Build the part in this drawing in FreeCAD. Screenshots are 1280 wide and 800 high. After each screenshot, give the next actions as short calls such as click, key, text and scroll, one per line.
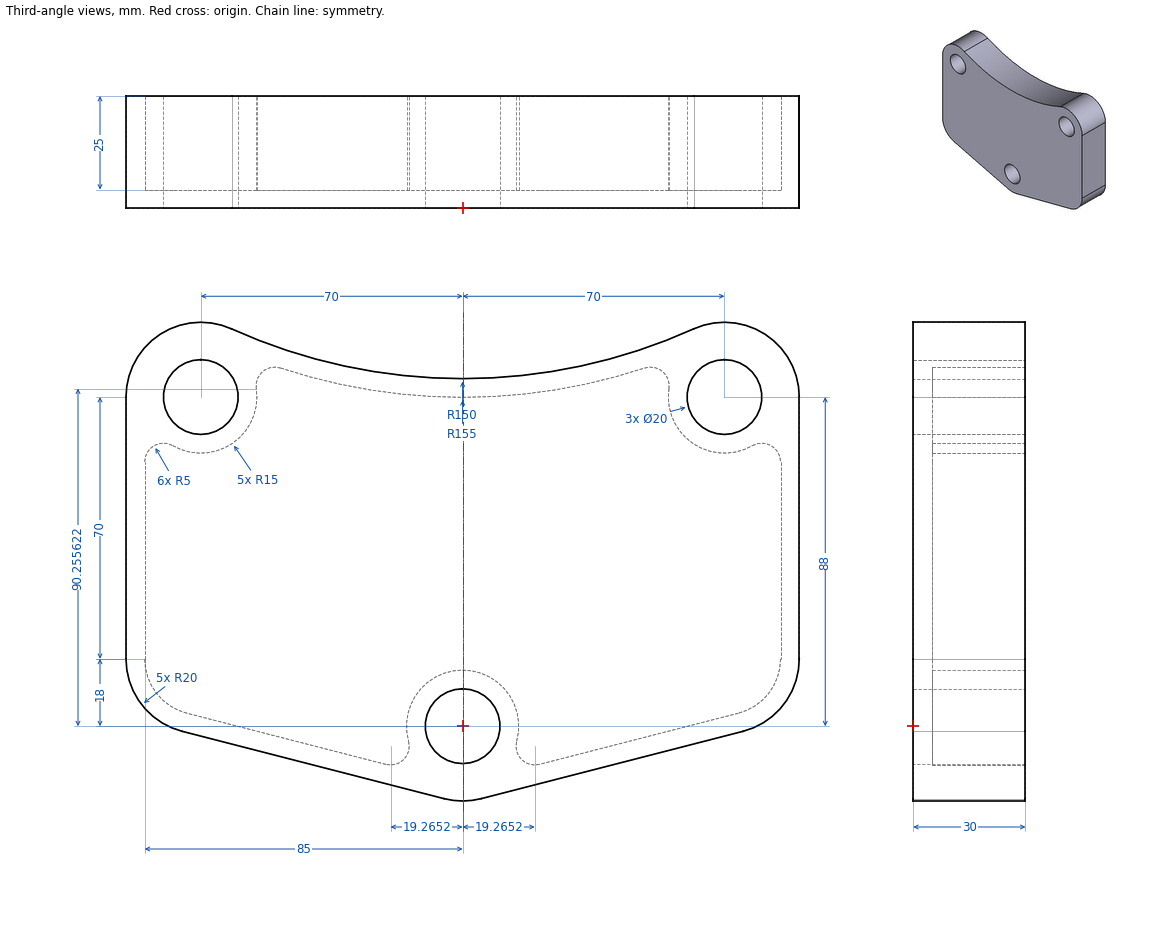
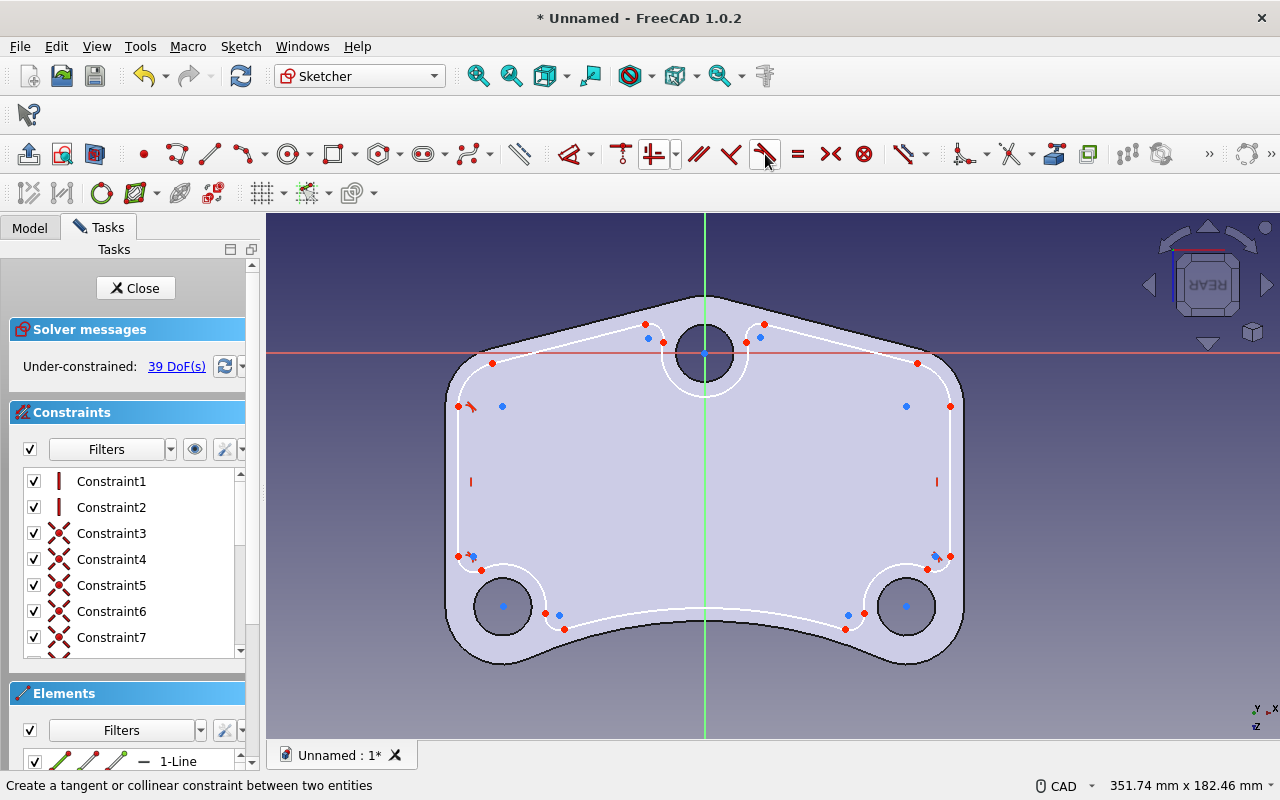
click(950, 512)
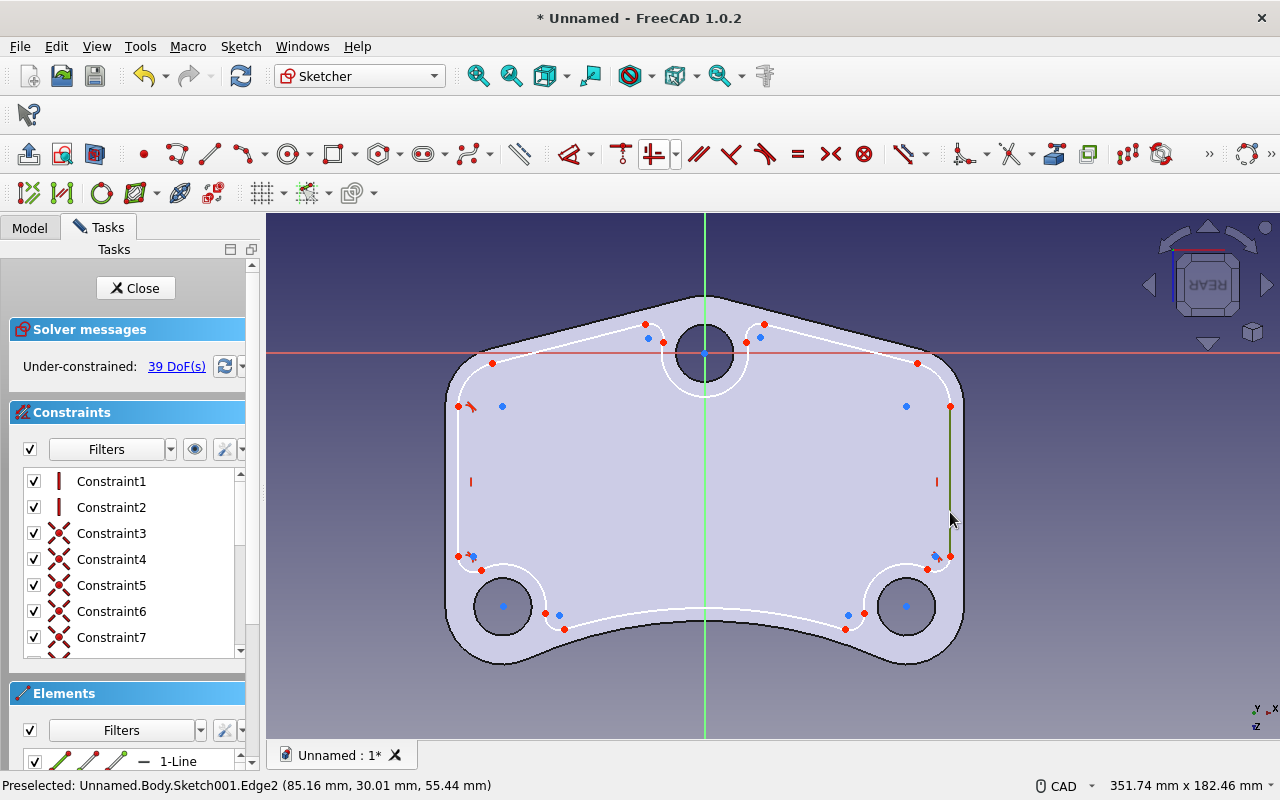
click(947, 390)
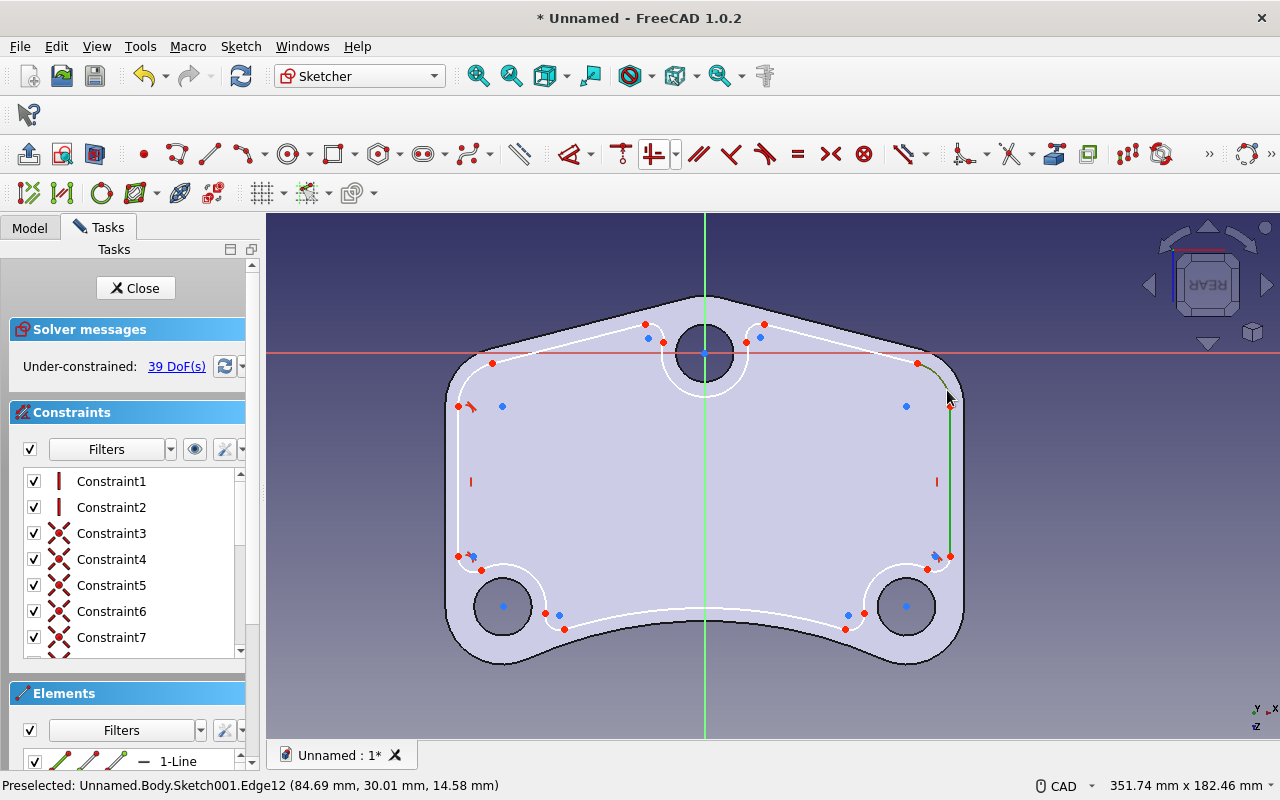
click(765, 154)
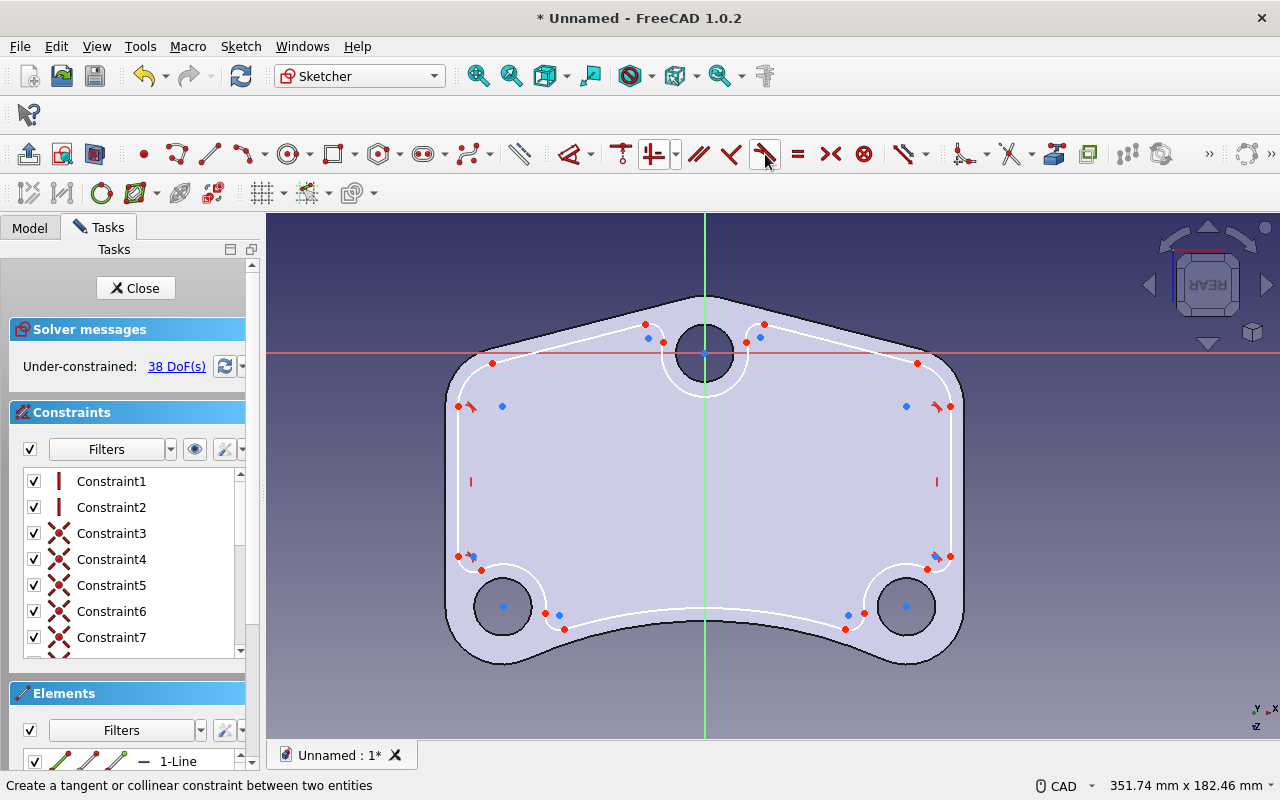
click(871, 352)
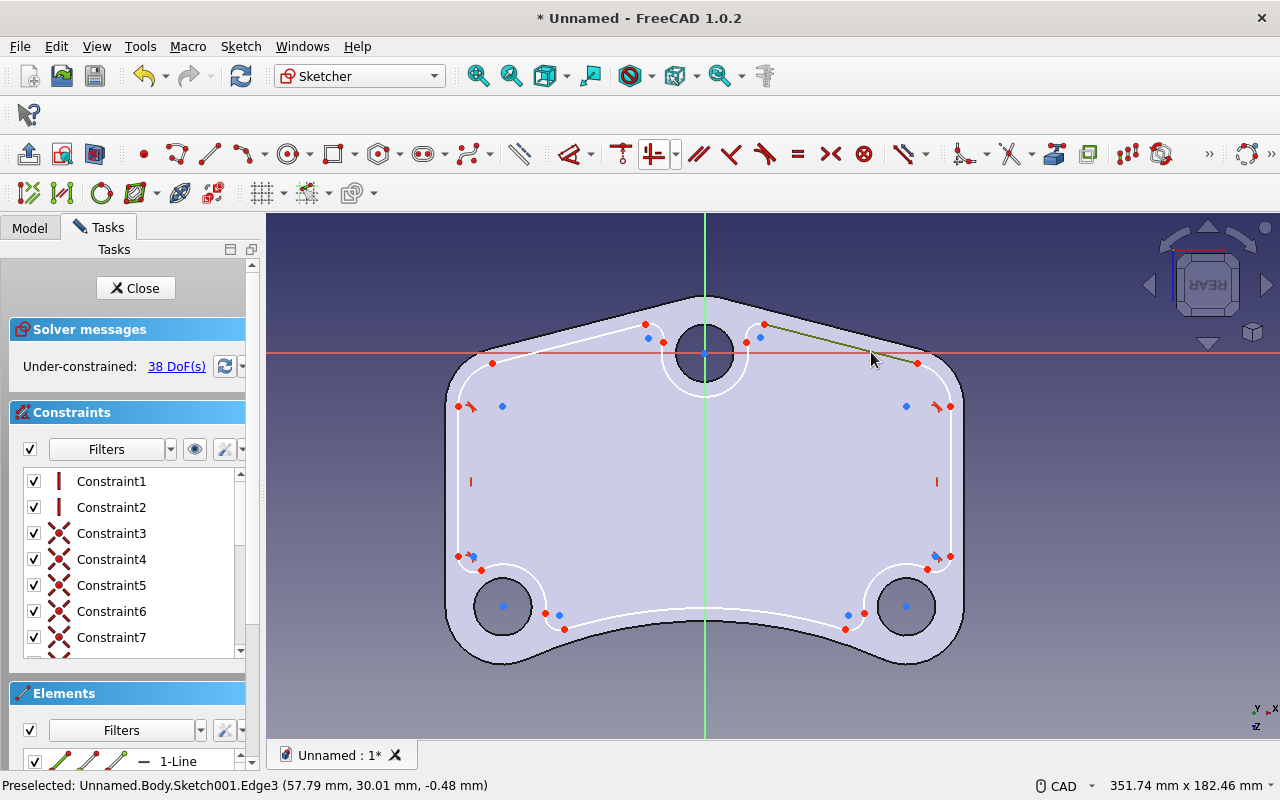
click(947, 390)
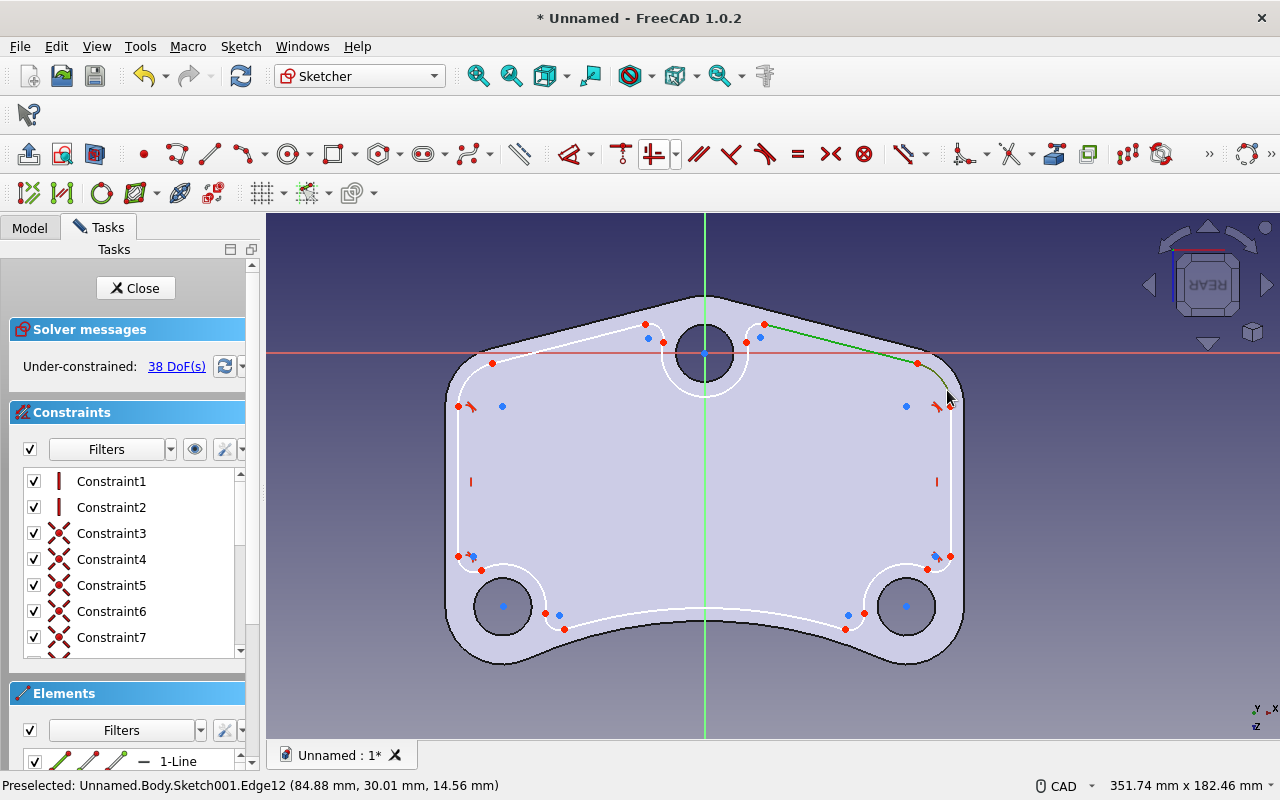
click(765, 154)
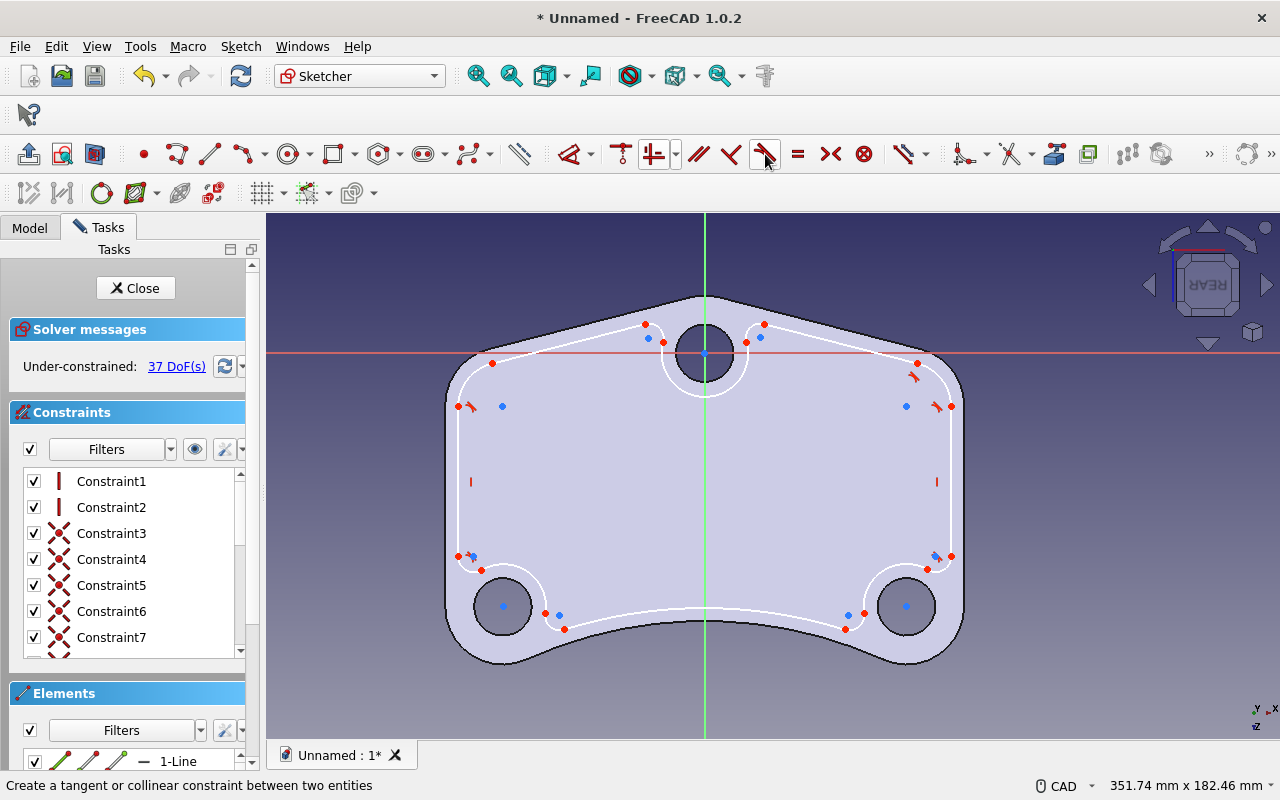
click(872, 352)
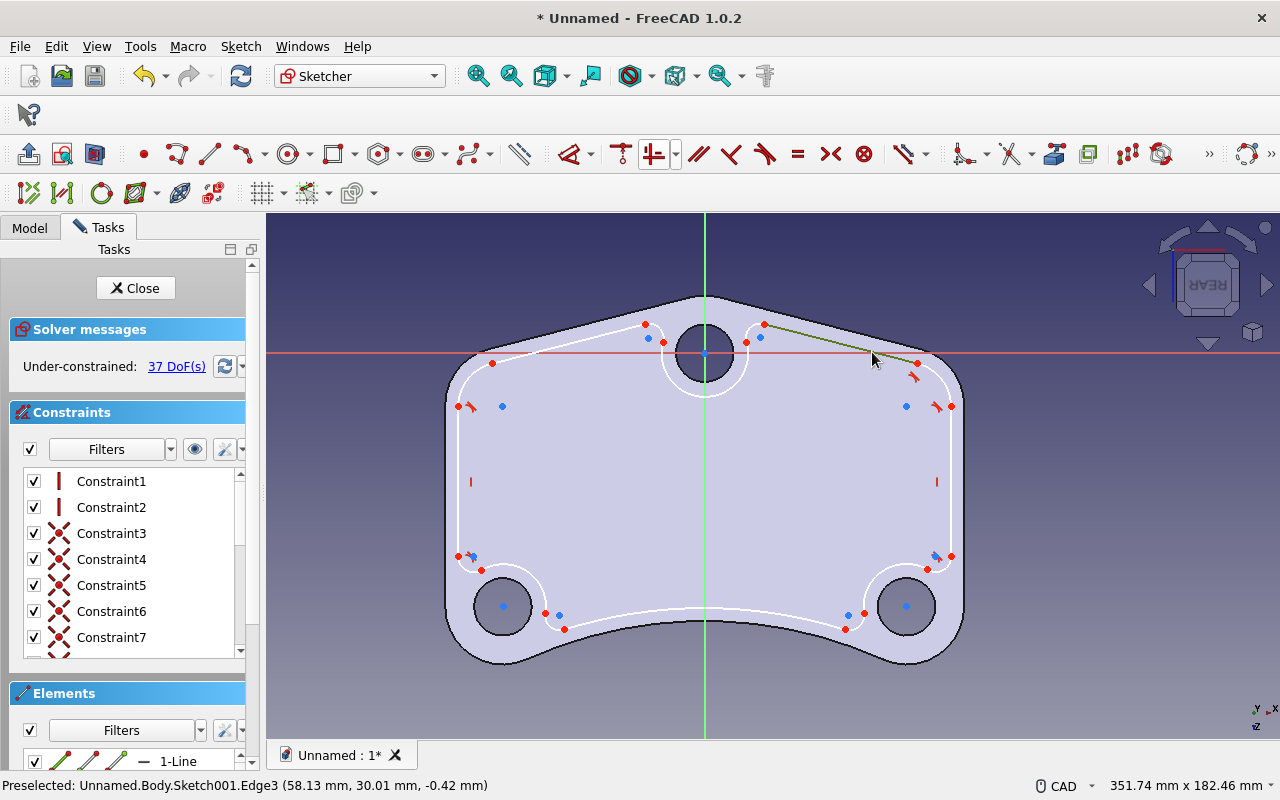
scroll(755, 325, up, 3)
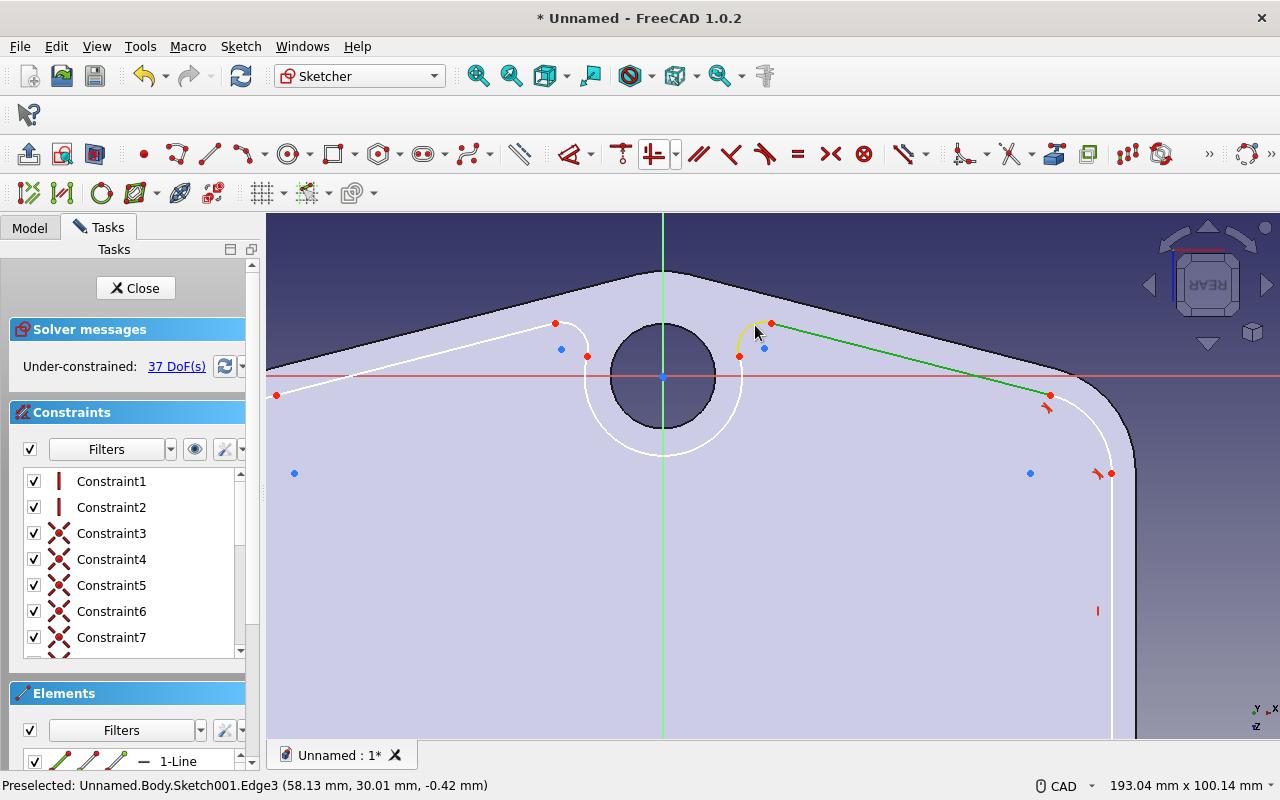
click(755, 324)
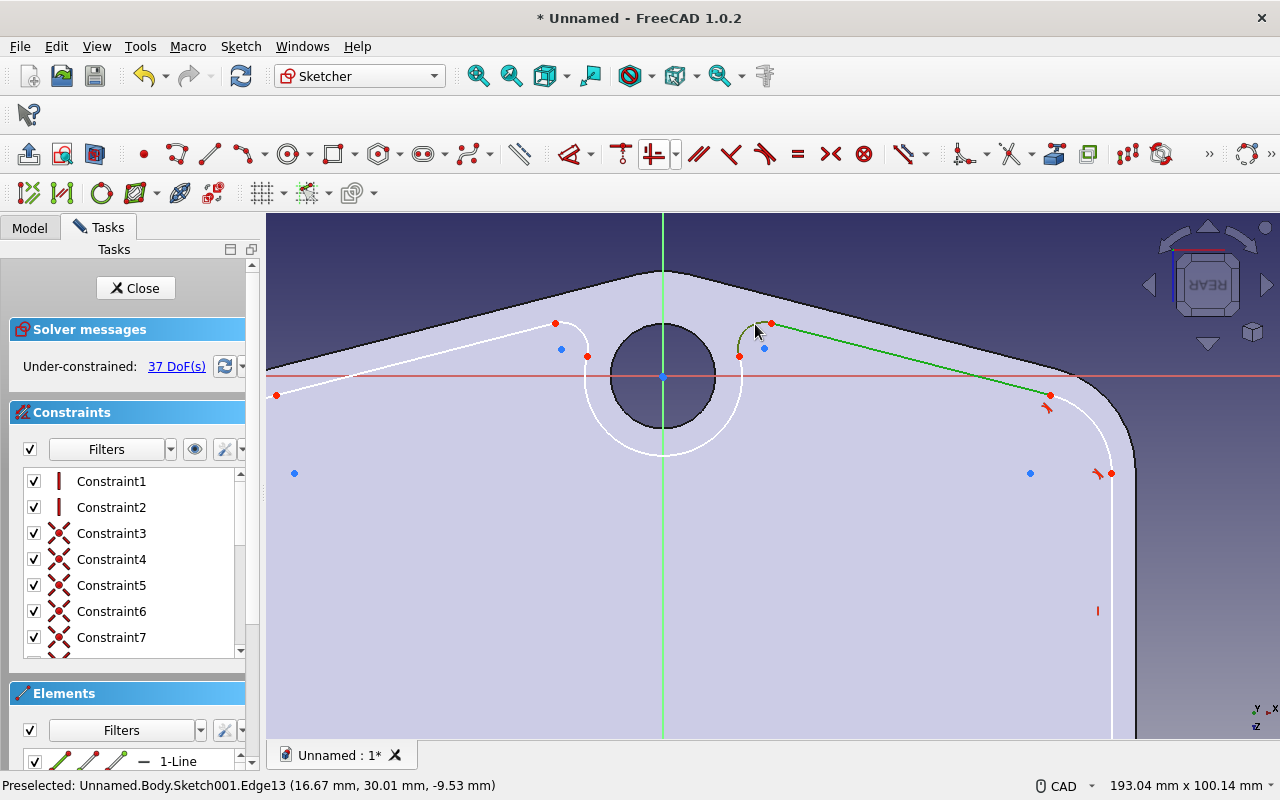
click(765, 154)